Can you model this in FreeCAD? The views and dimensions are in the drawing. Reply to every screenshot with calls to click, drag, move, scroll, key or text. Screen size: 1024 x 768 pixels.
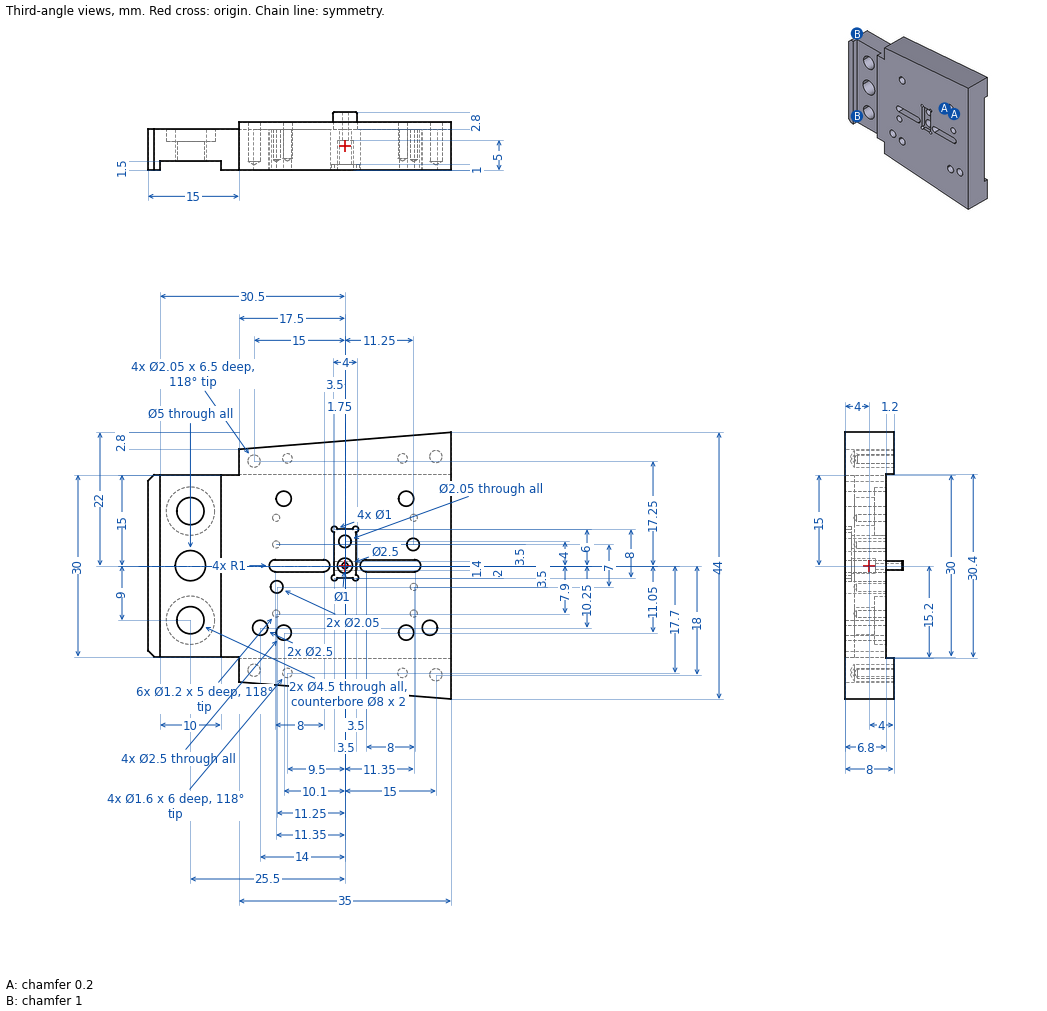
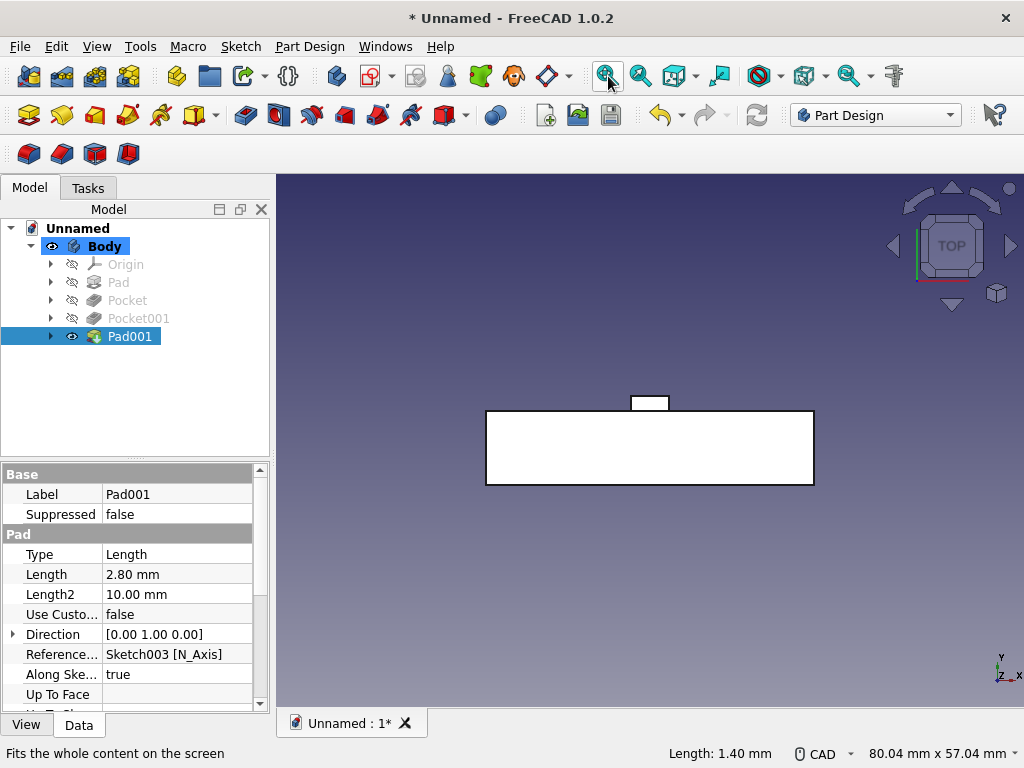
scroll(669, 395, up, 6)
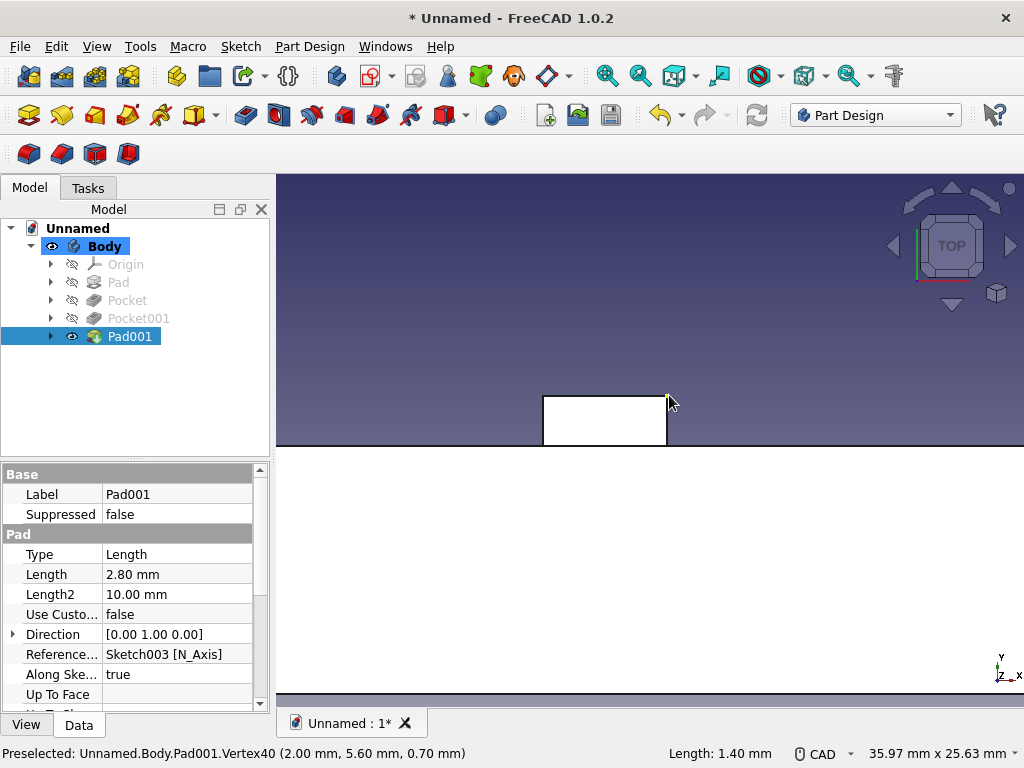
click(608, 76)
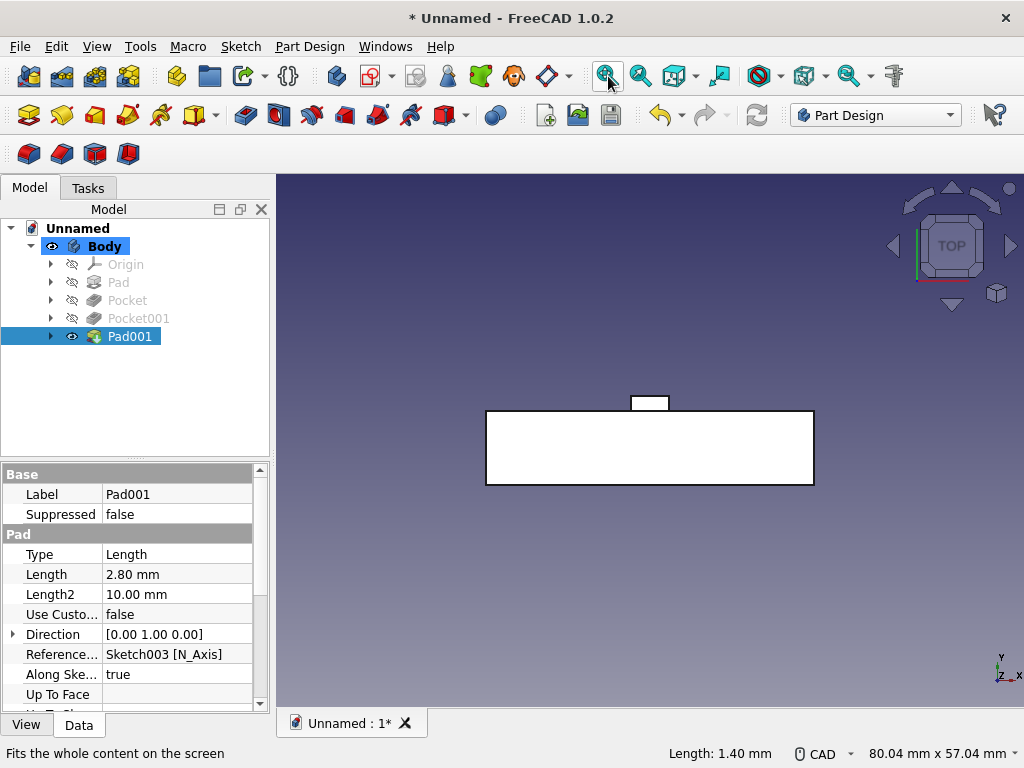
key(1)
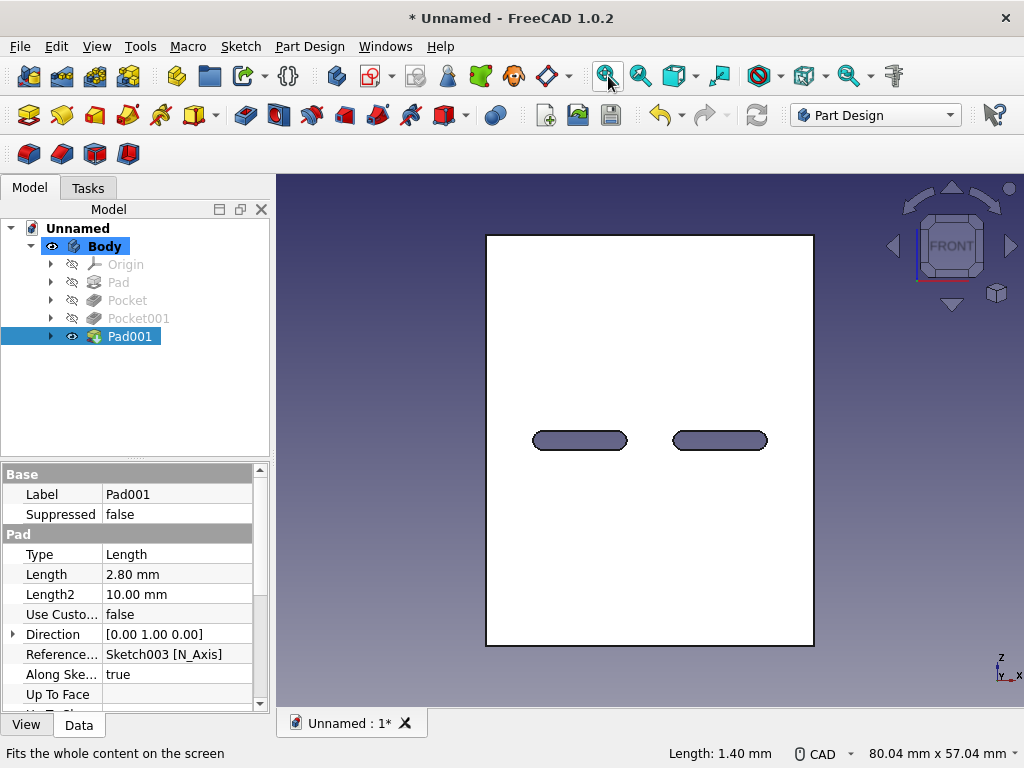
scroll(669, 440, up, 6)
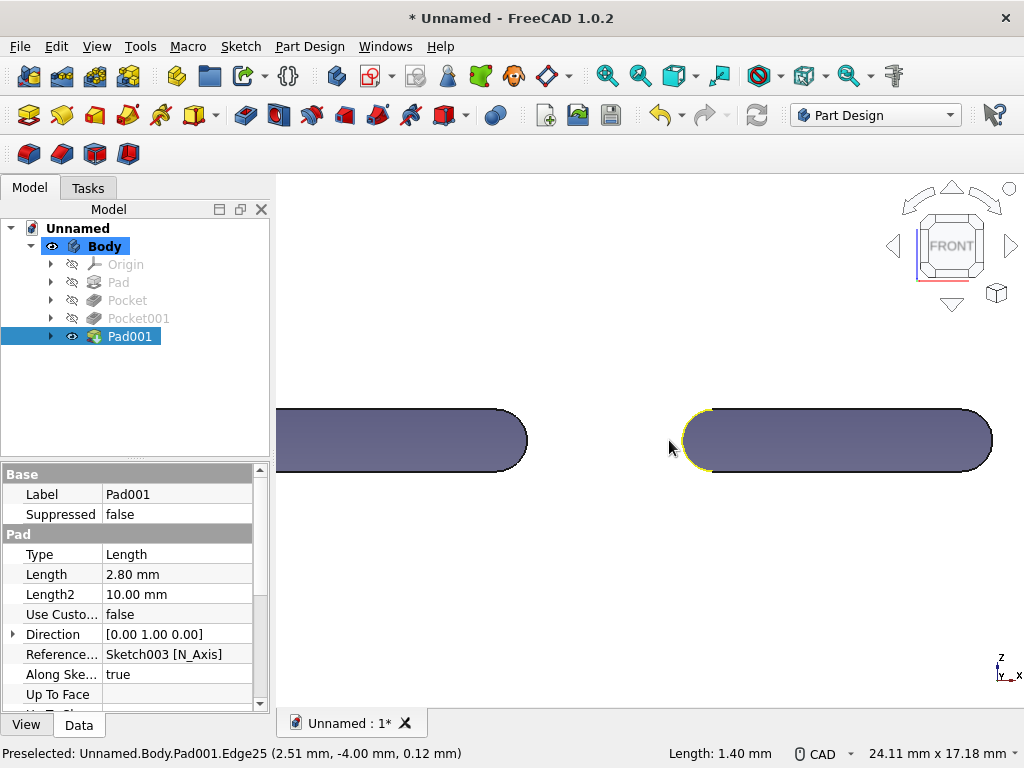
click(608, 76)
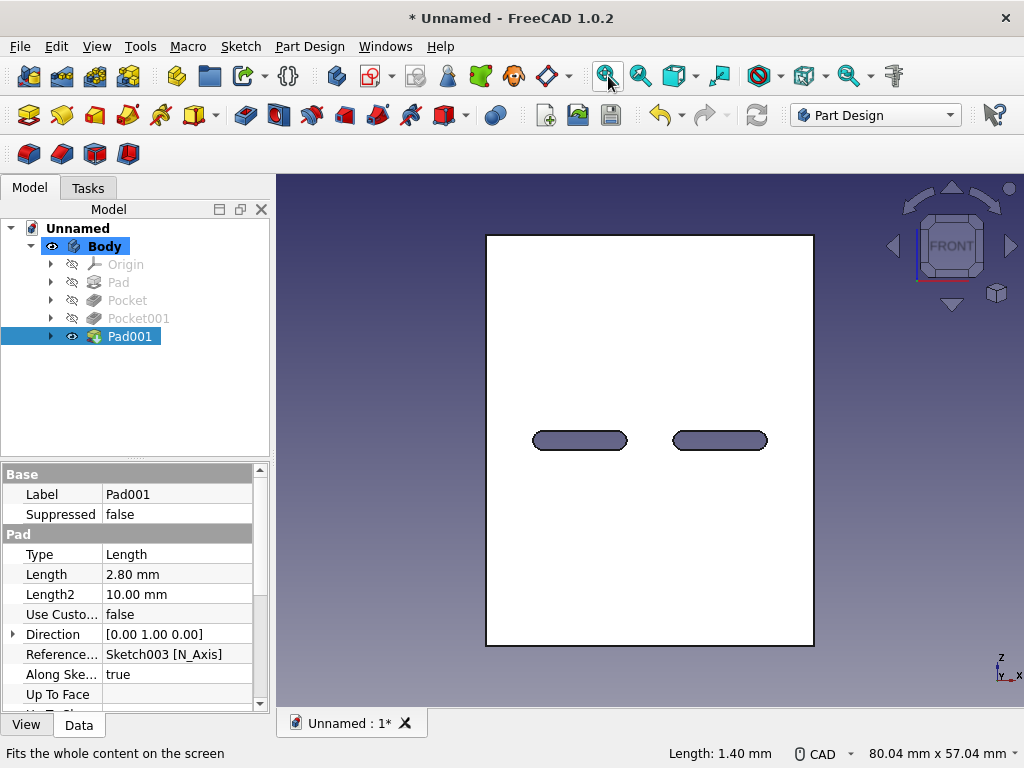
key(3)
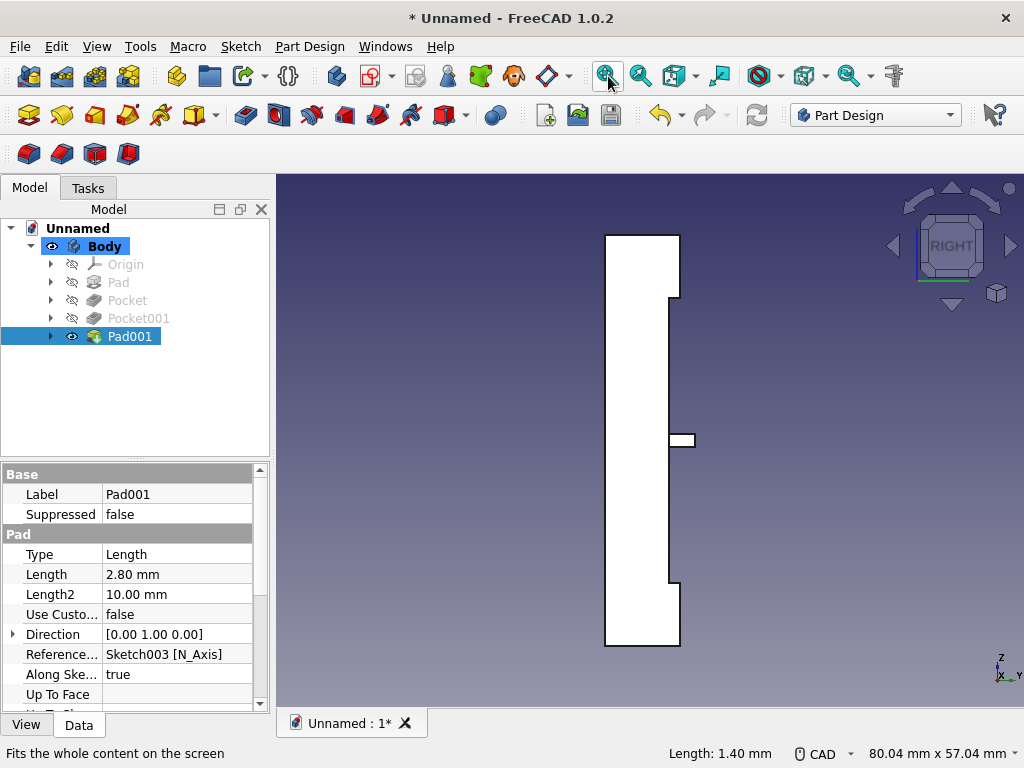
click(695, 439, ctrl)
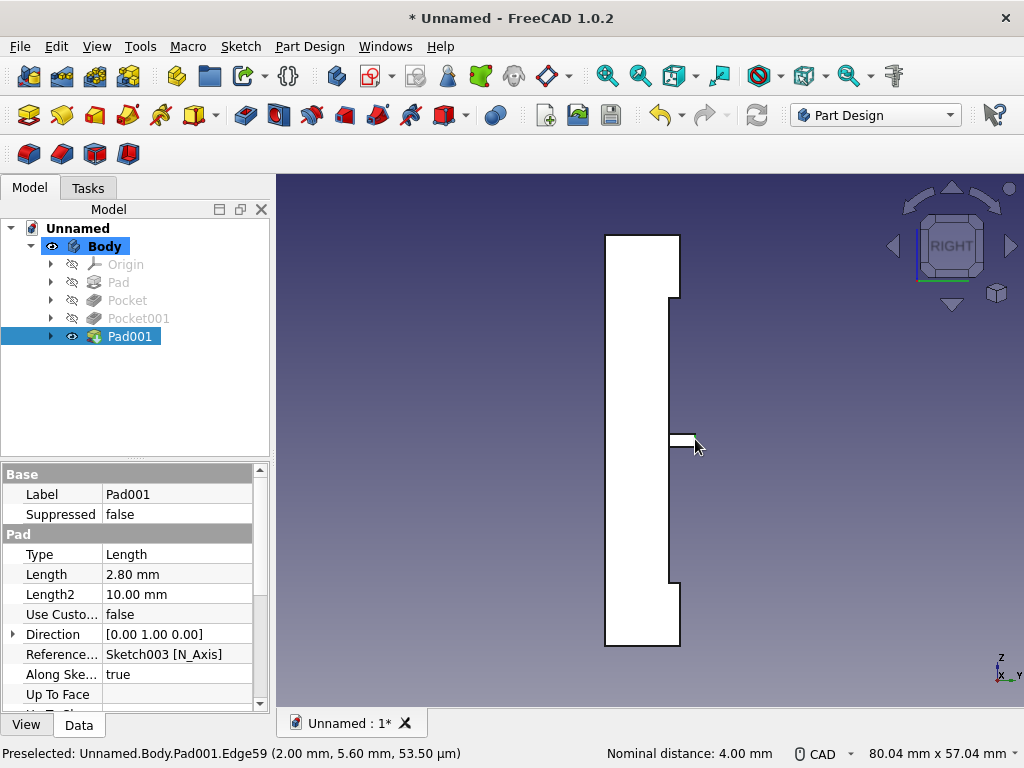
click(62, 154)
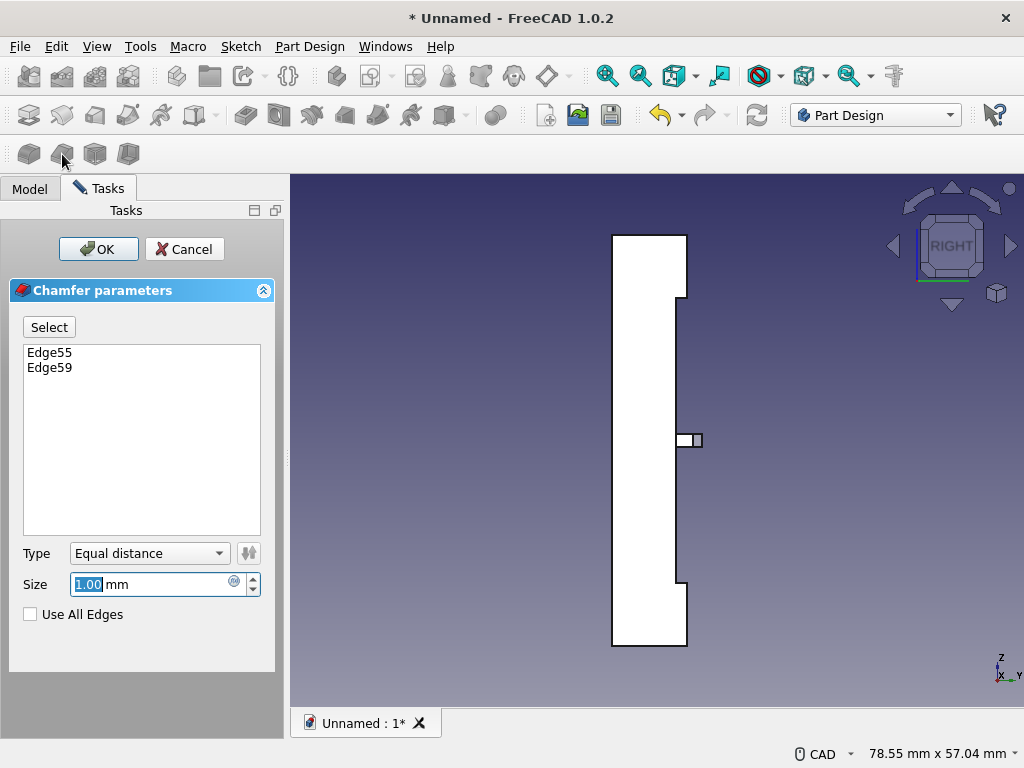
text(0.2)
key(Tab)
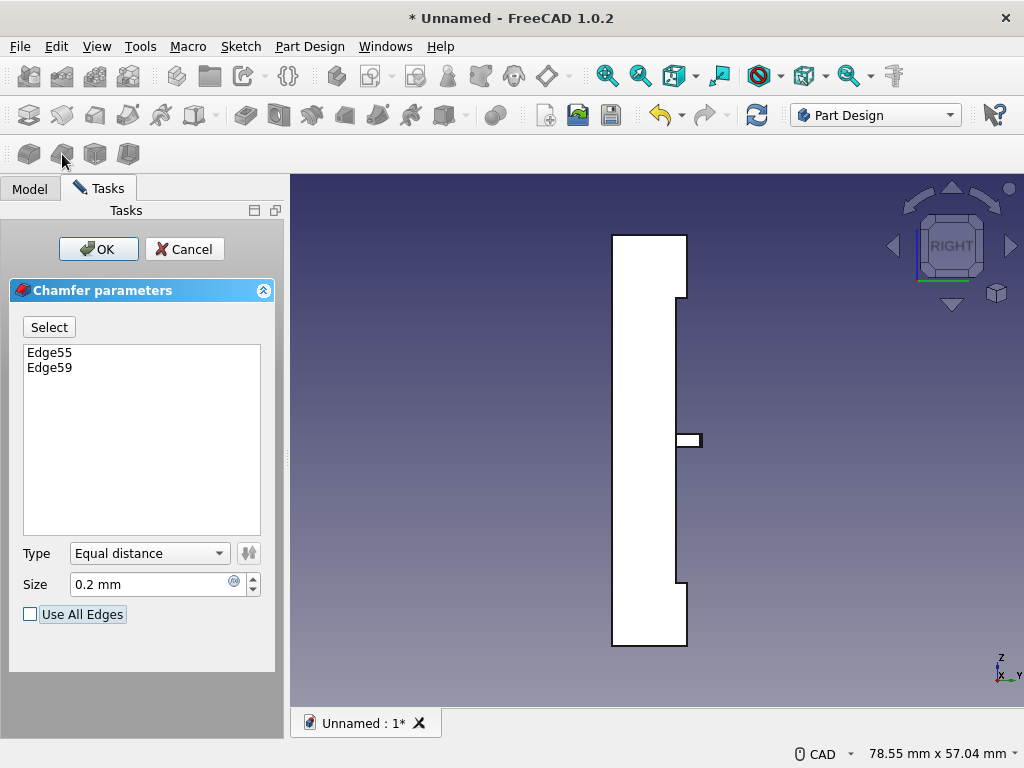
click(99, 249)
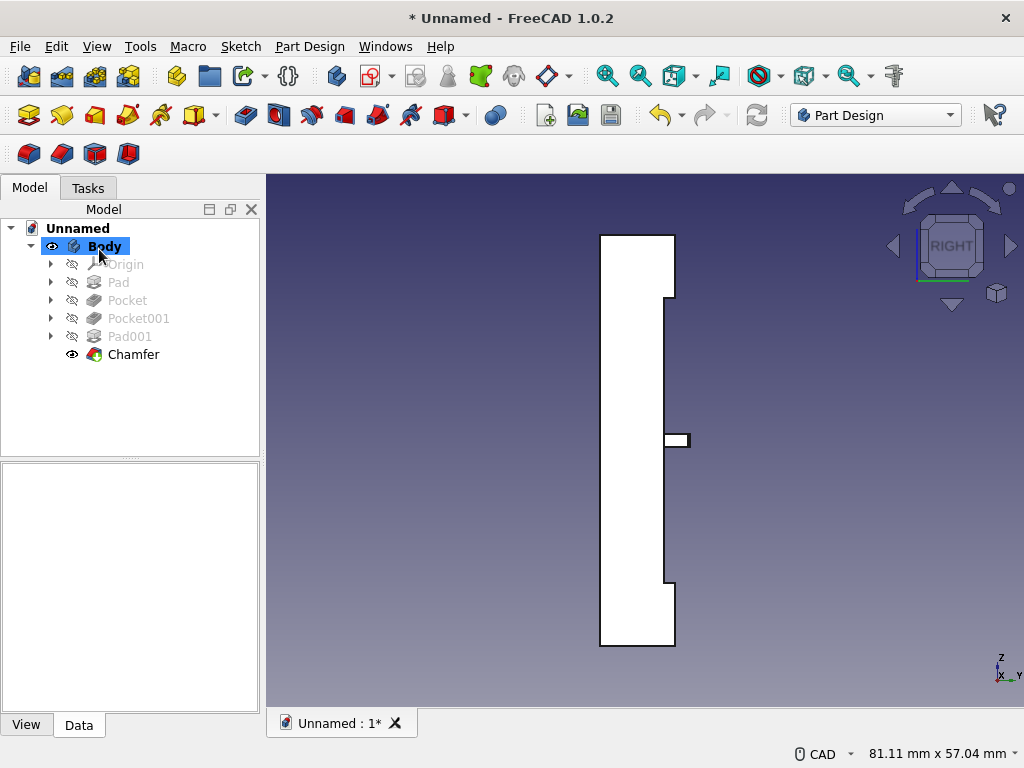
key(0)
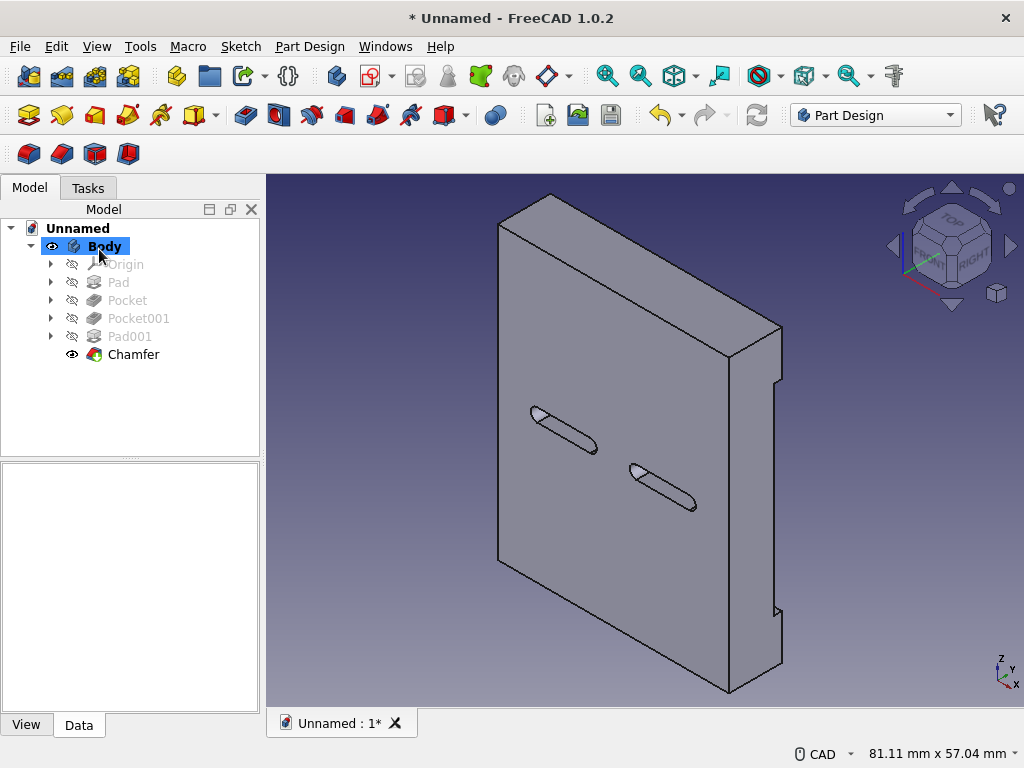
click(646, 573)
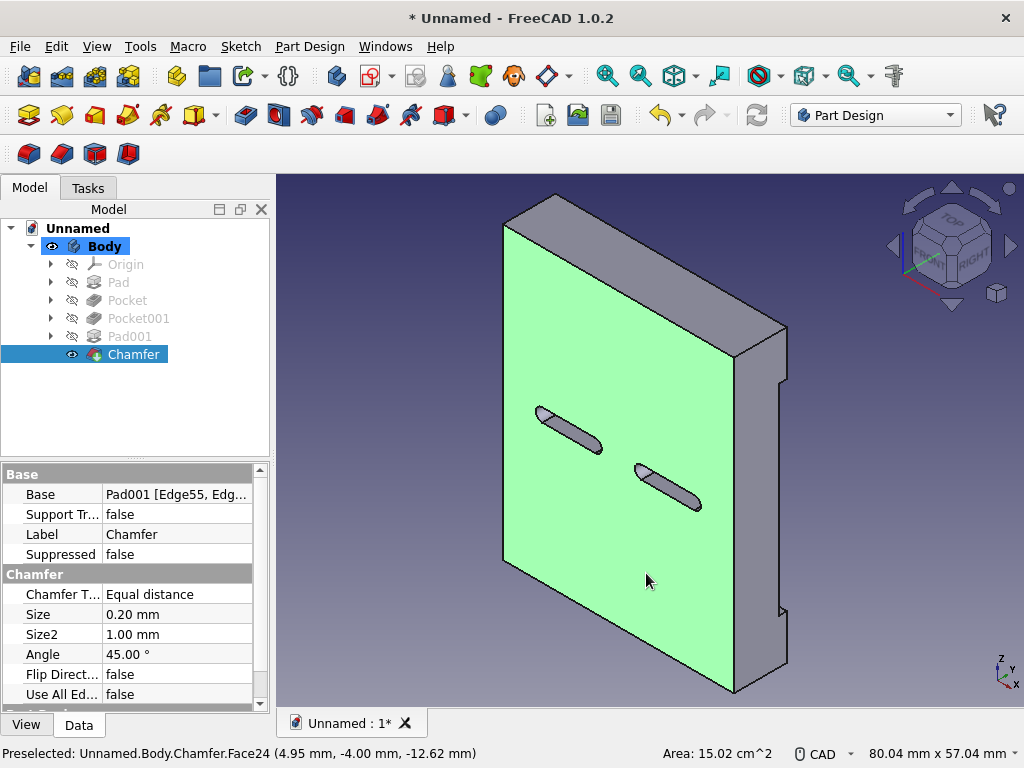
click(370, 76)